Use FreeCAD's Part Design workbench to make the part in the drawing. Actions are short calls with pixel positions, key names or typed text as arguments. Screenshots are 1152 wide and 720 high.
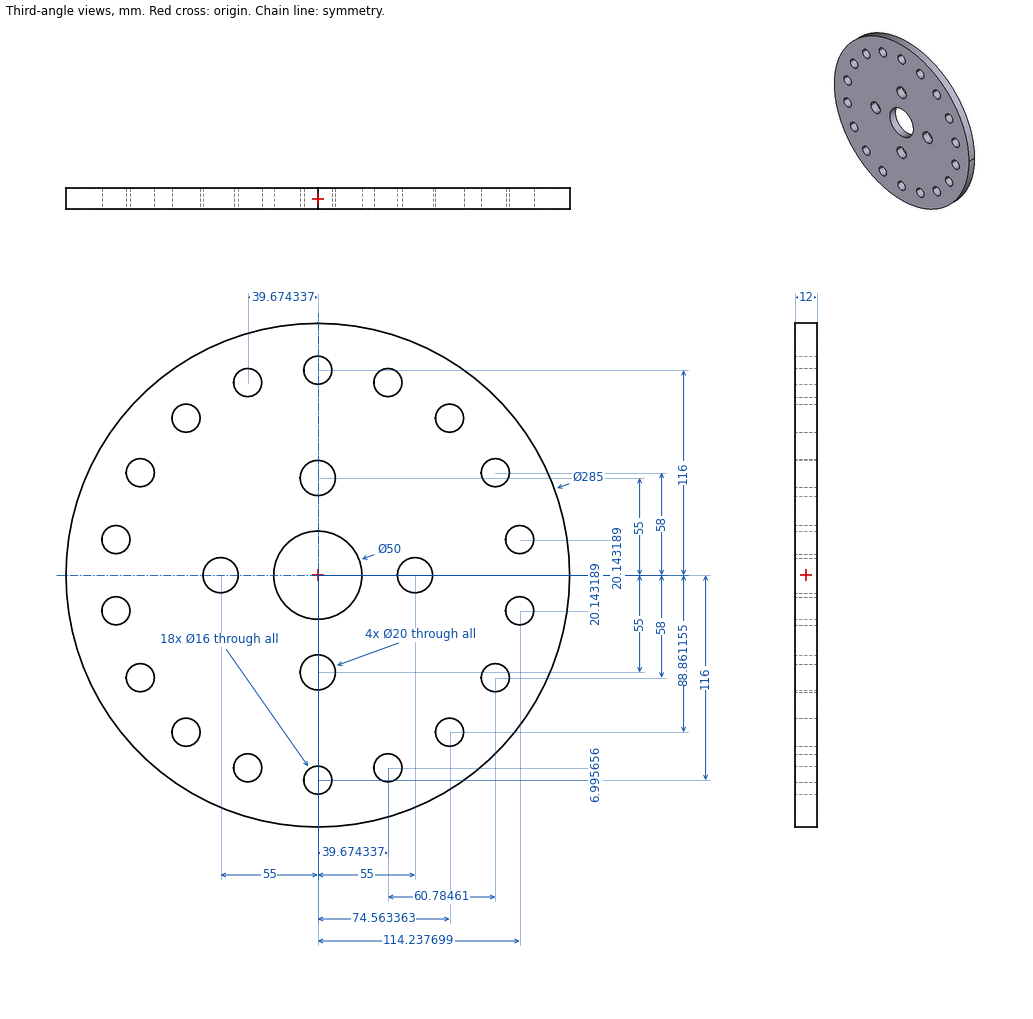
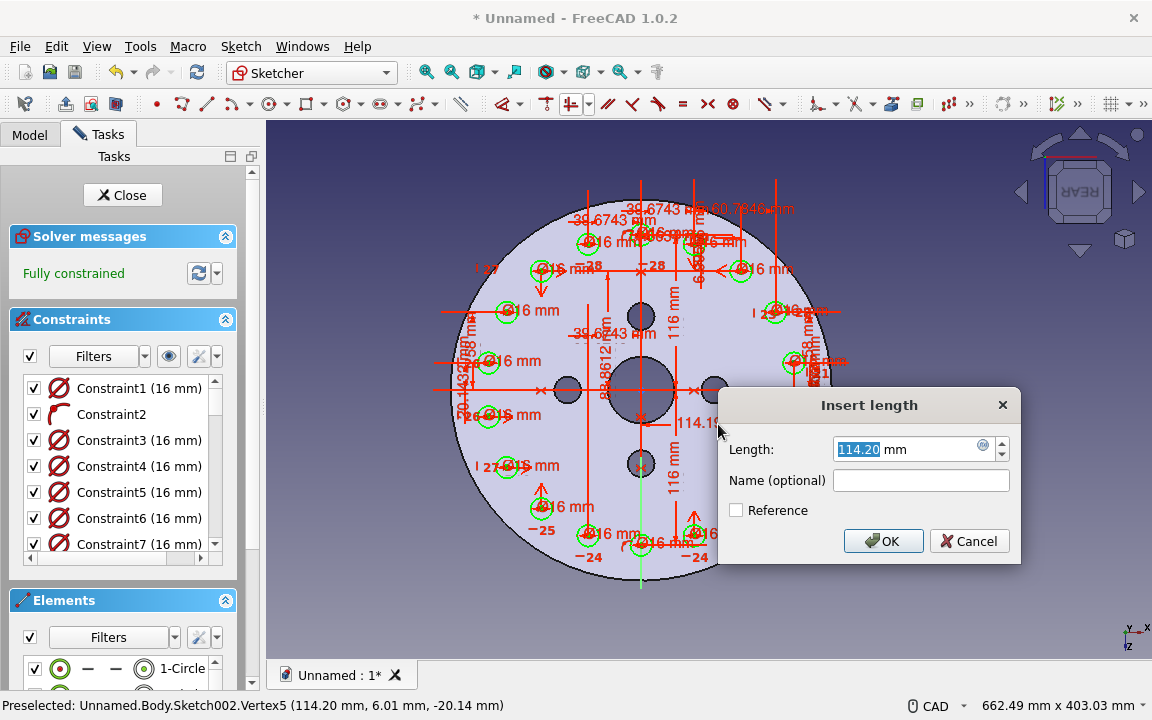
text(114.237699)
key(Return)
key(Escape)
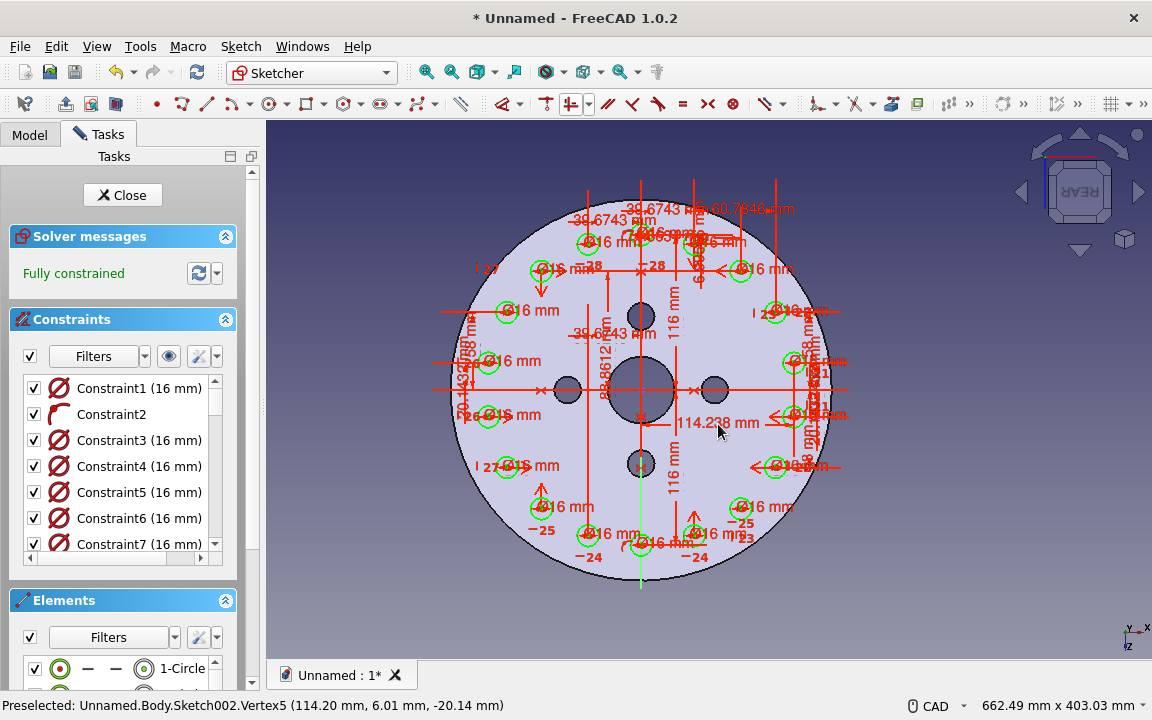
click(123, 195)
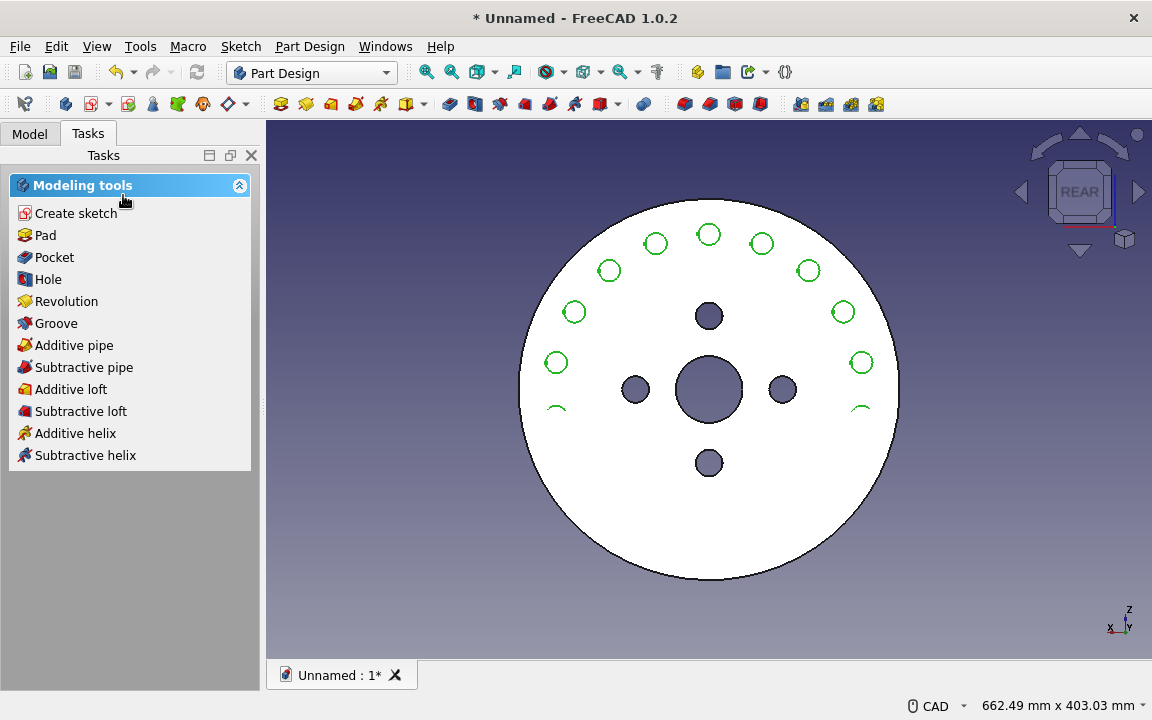
click(475, 104)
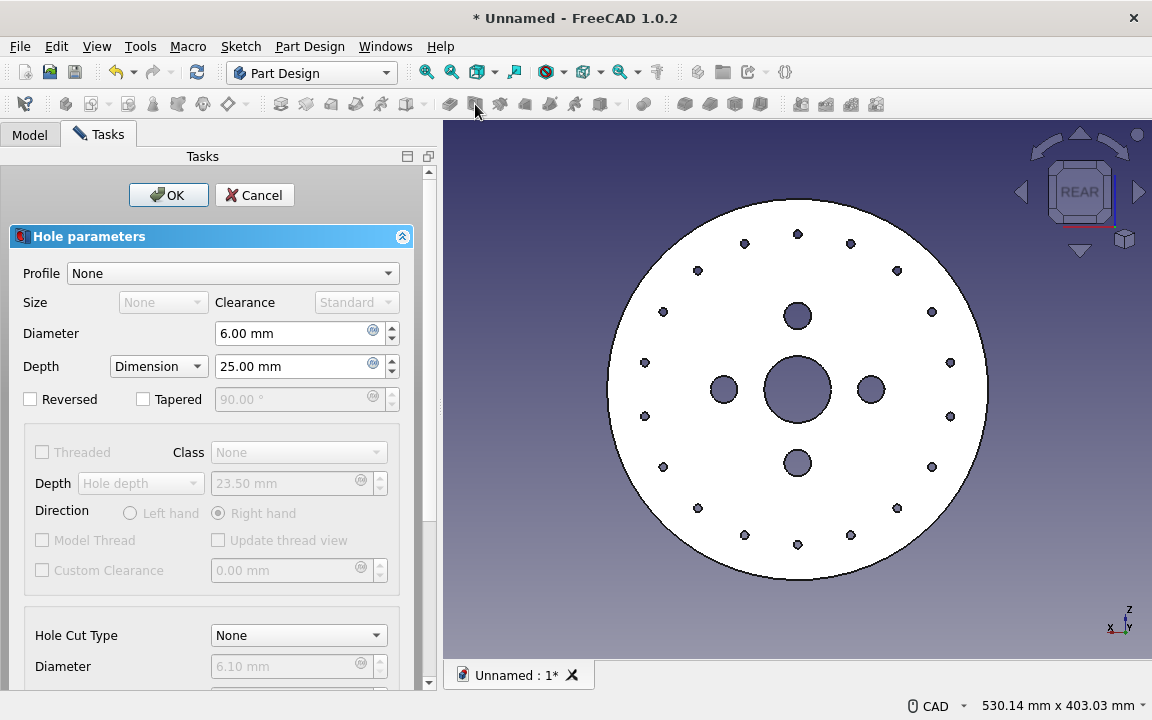
triple_click(300, 334)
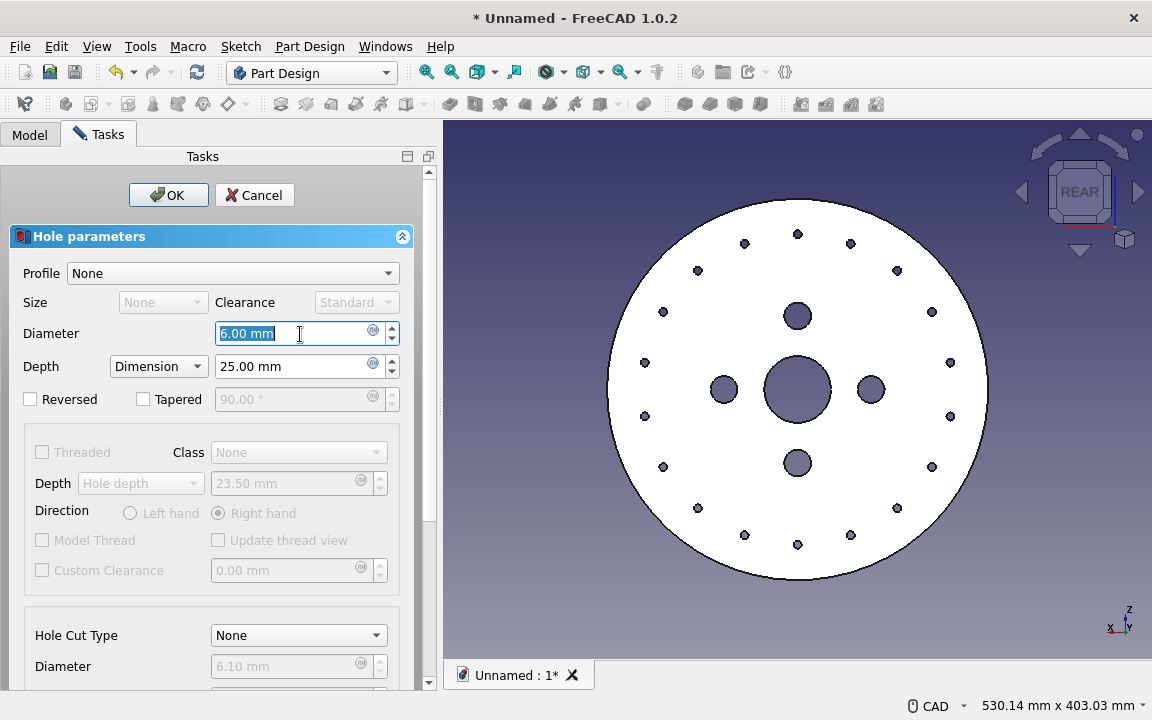
text(16)
key(Tab)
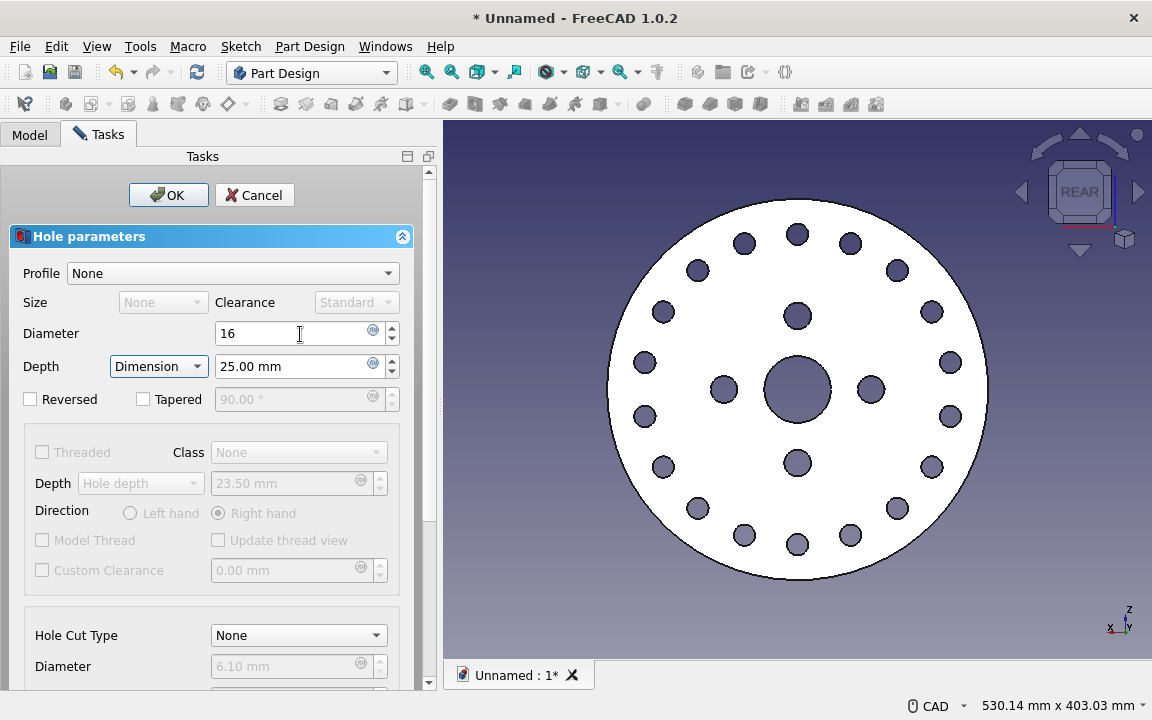
click(160, 366)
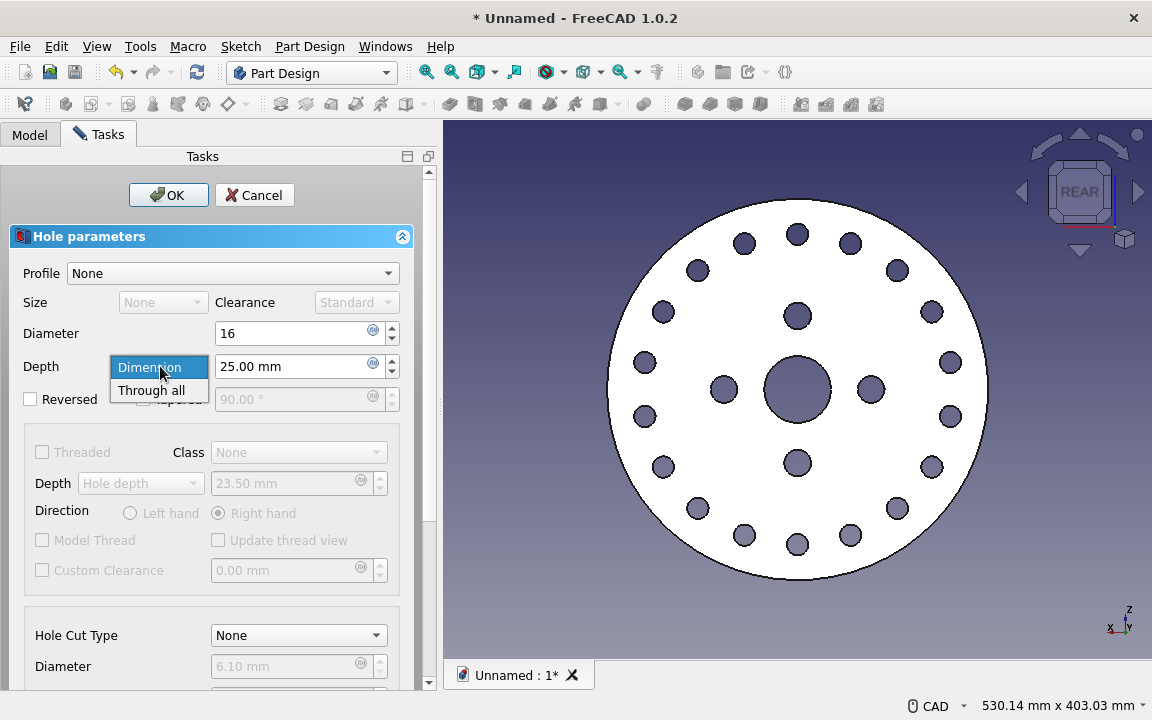
click(158, 390)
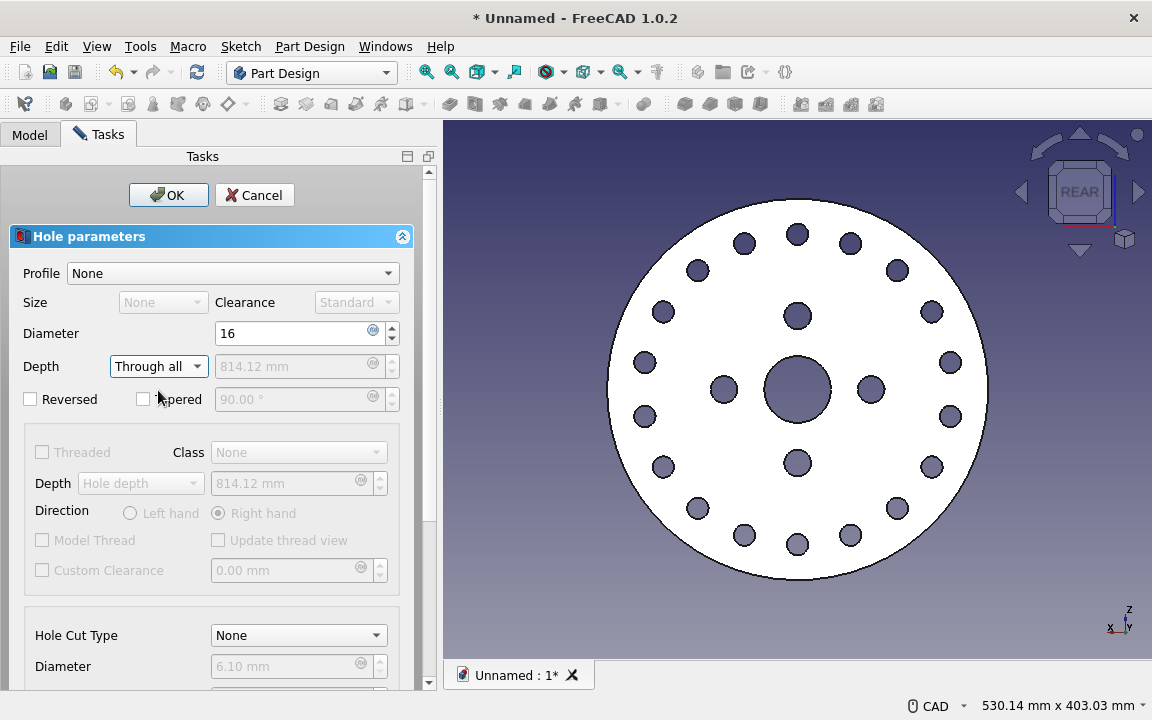
click(169, 195)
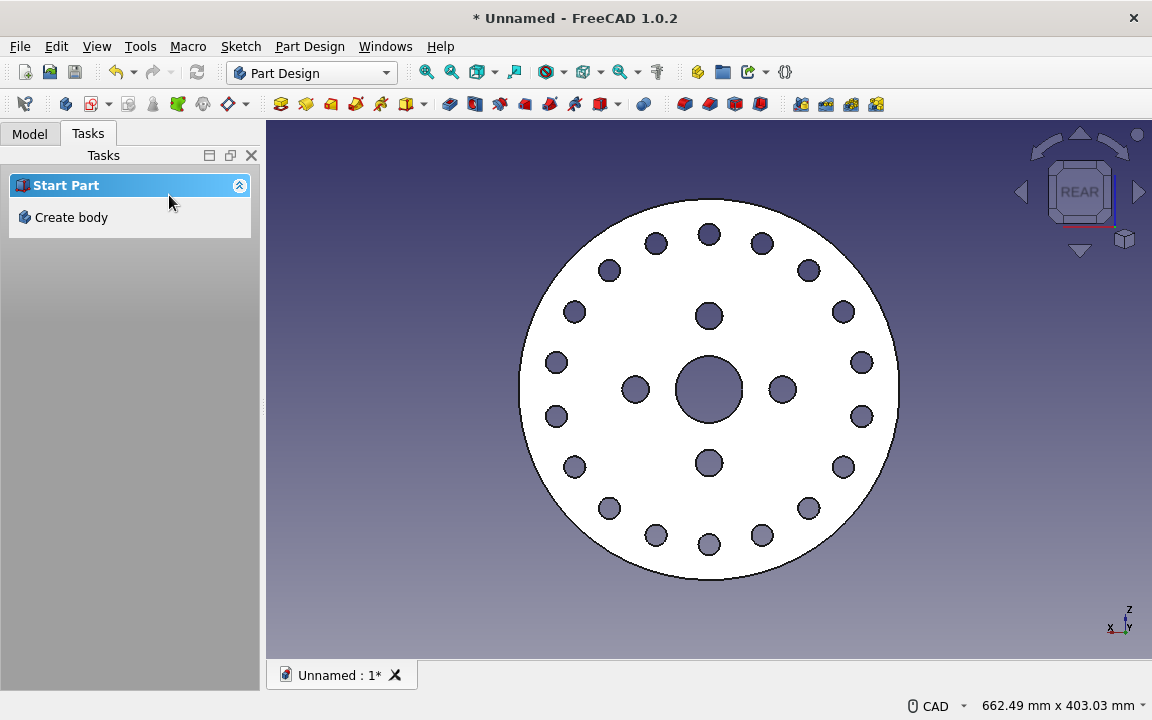
key(0)